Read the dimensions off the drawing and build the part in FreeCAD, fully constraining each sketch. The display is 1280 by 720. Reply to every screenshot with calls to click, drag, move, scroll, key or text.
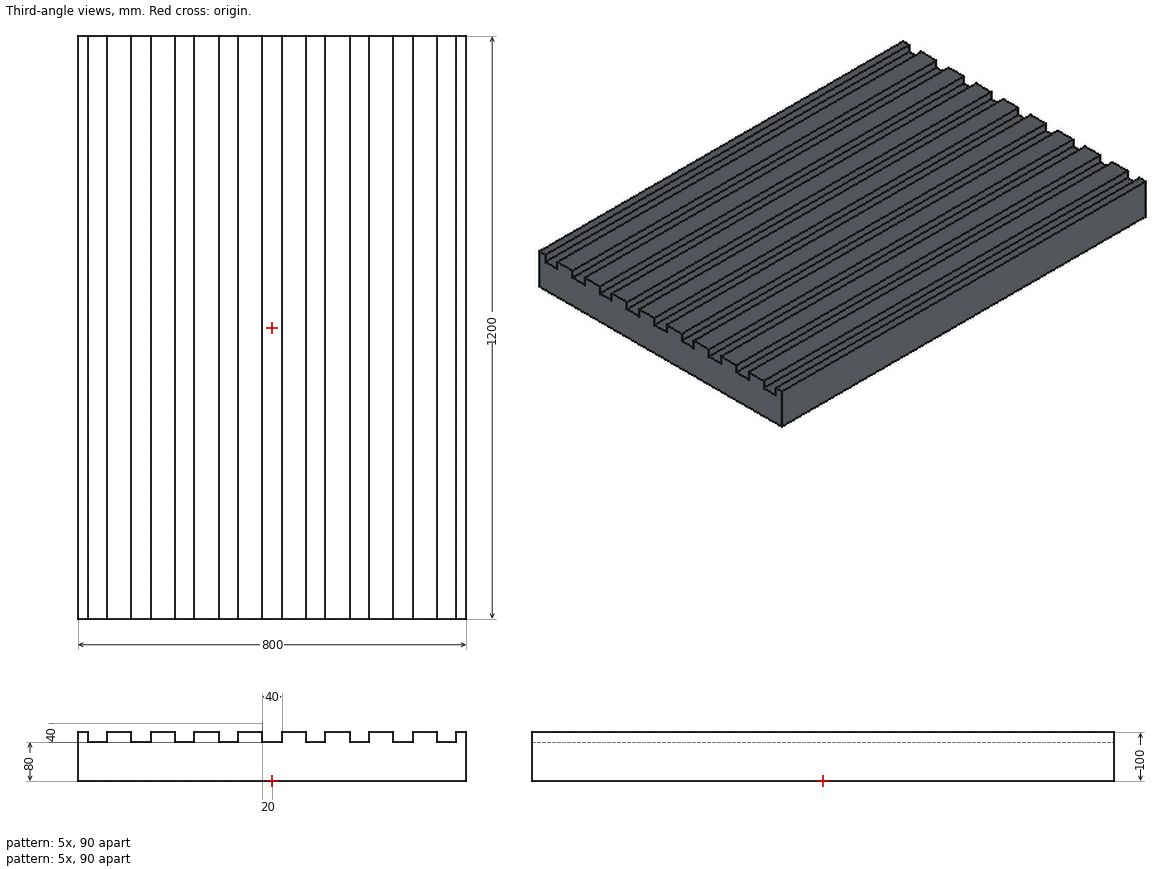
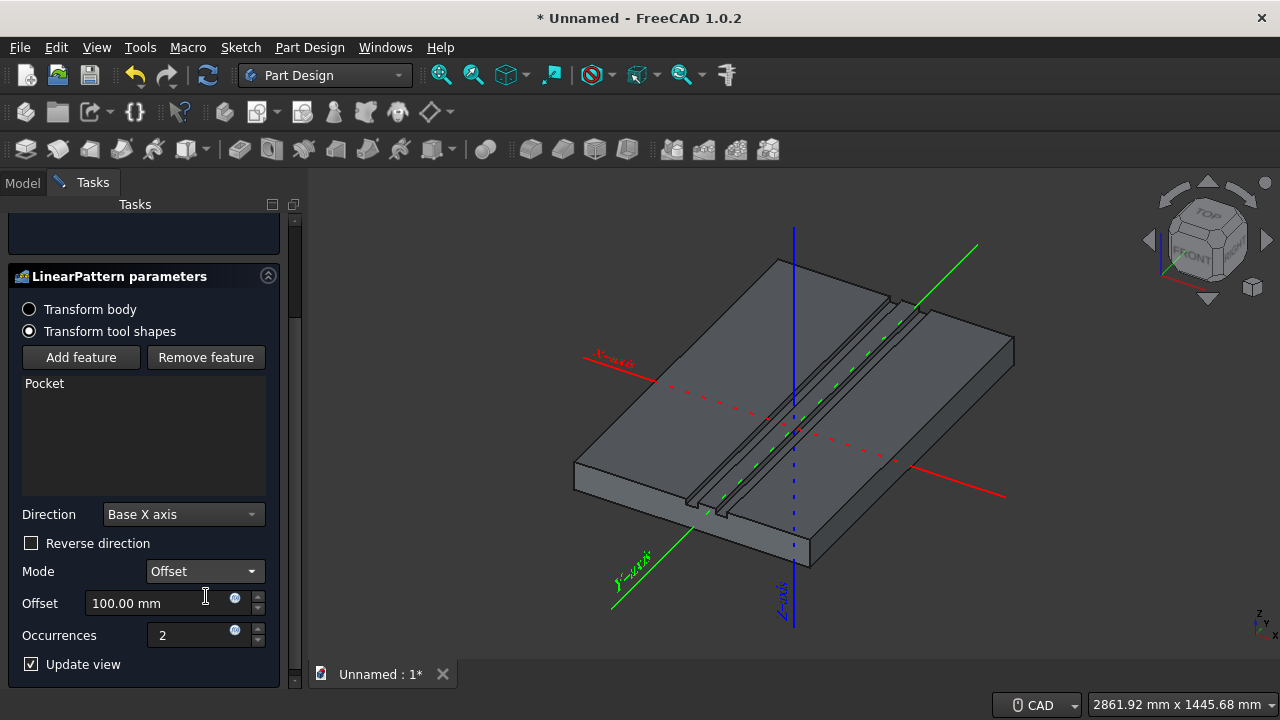
triple_click(168, 603)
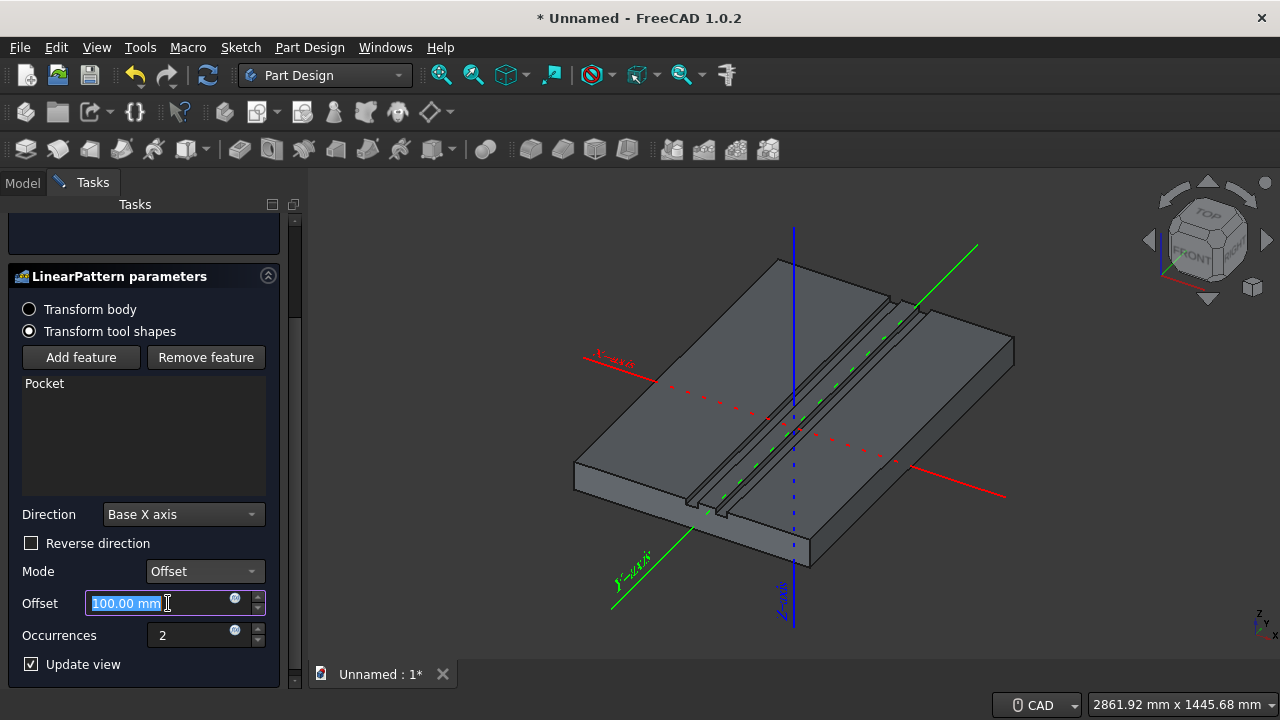
text(90)
key(Tab)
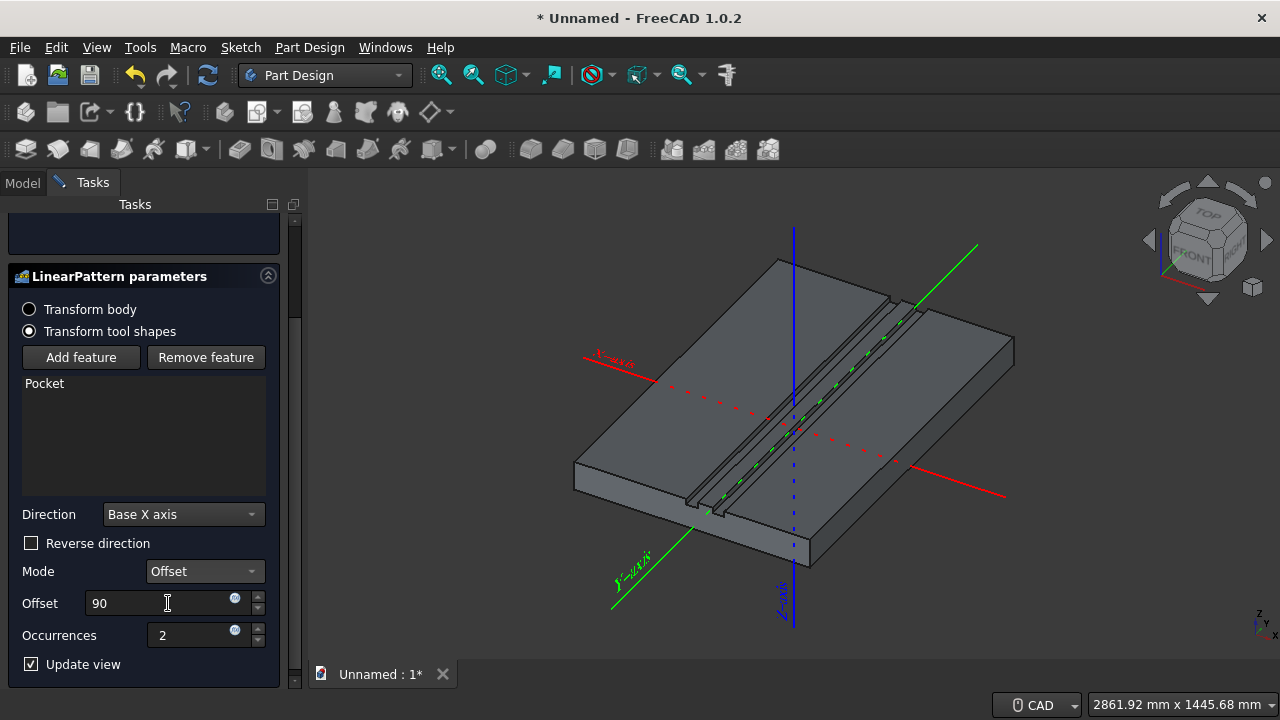
triple_click(198, 635)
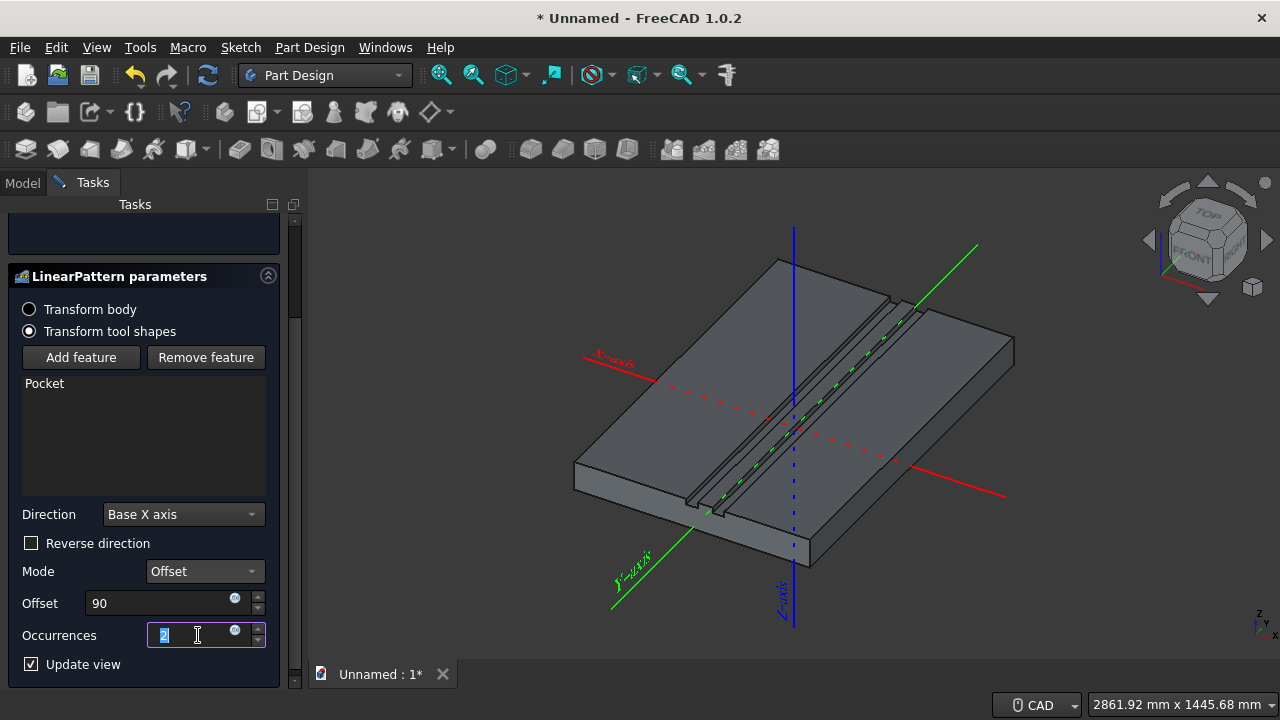
text(5)
key(Tab)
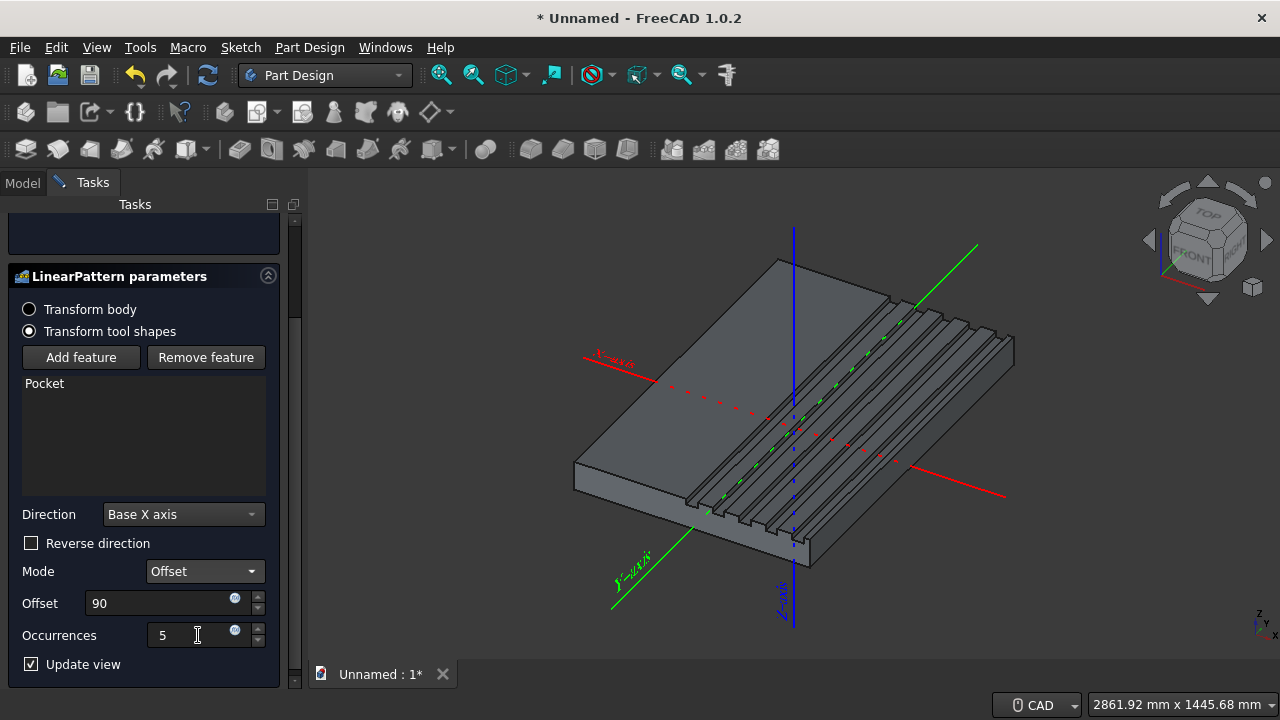
scroll(295, 451, up, 3)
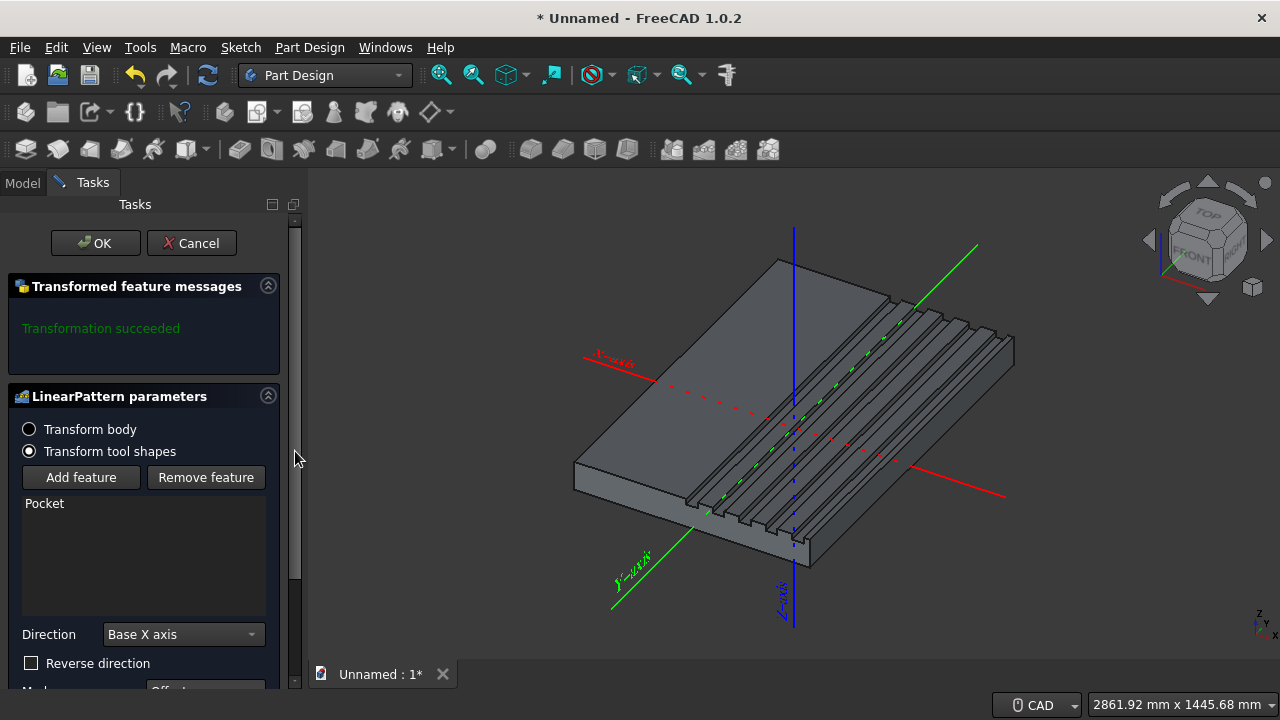
click(96, 243)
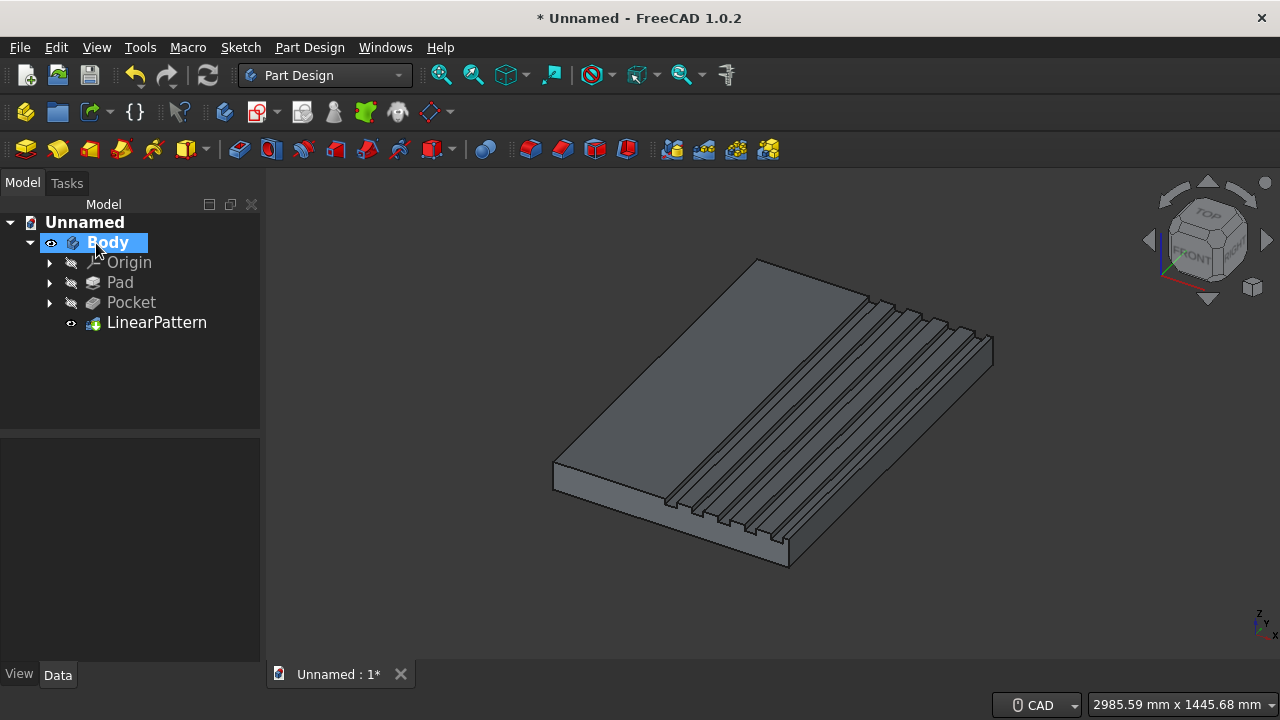
click(116, 303)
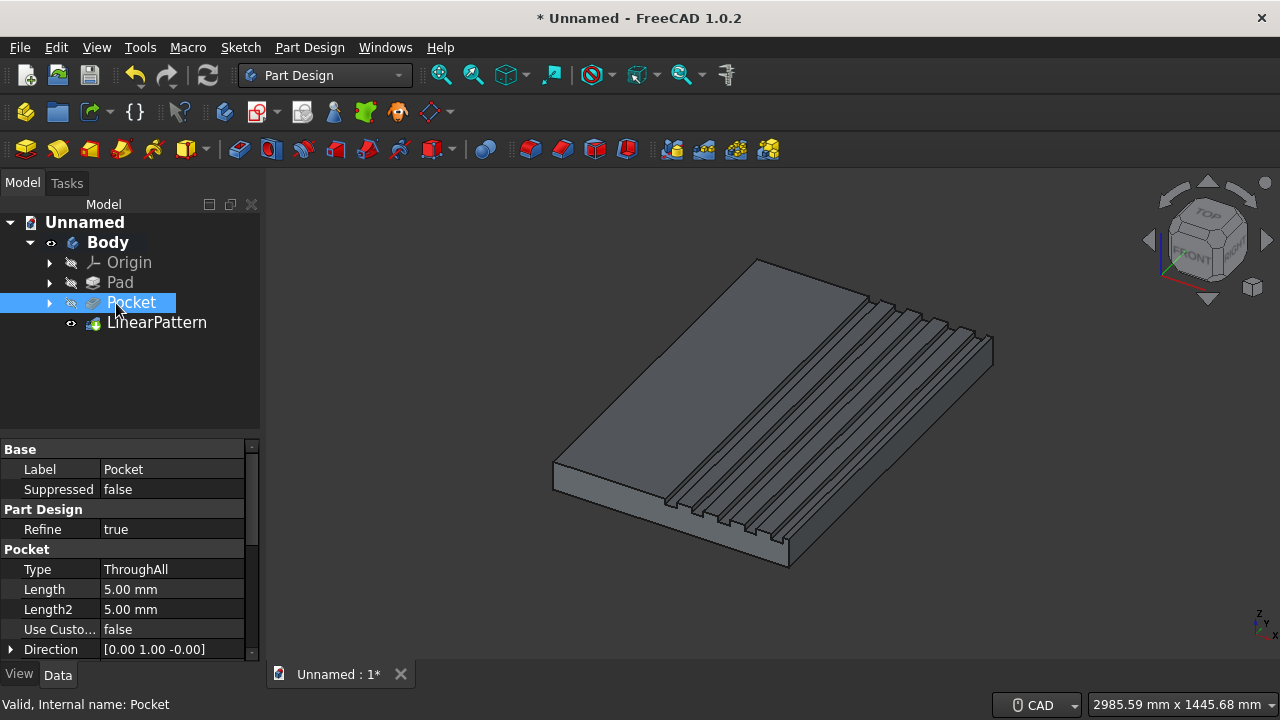
click(704, 150)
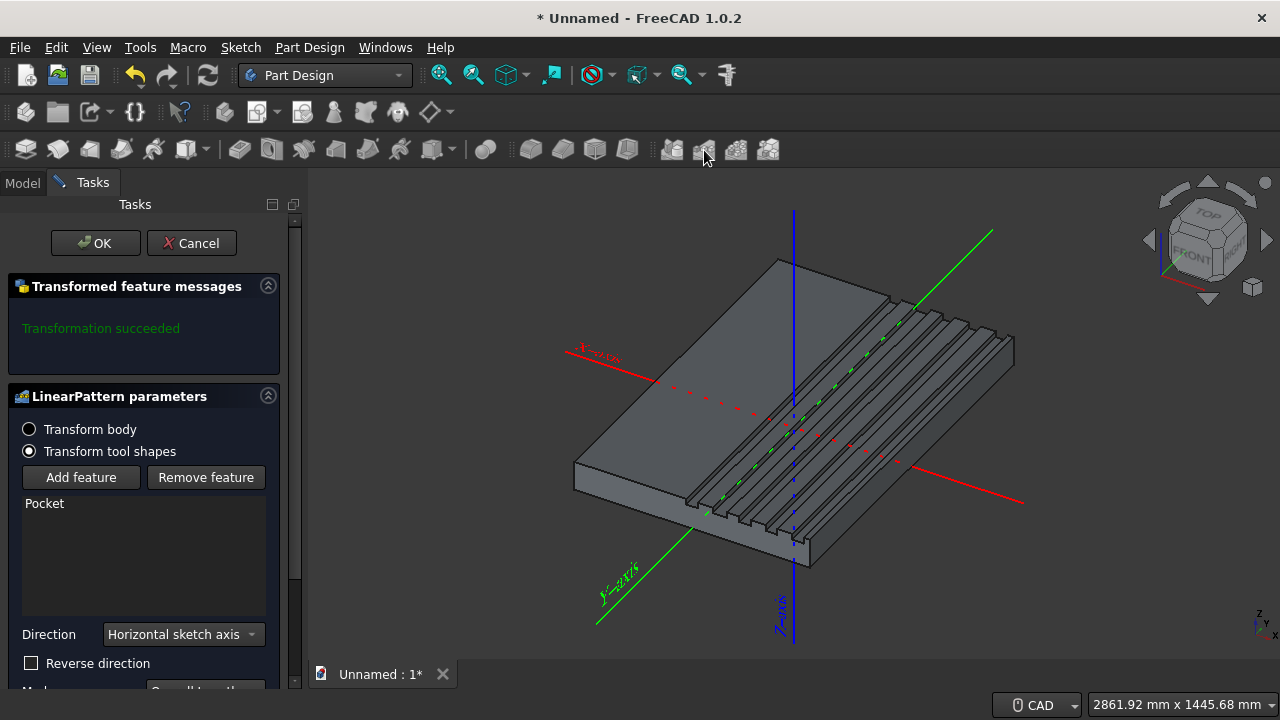
click(184, 634)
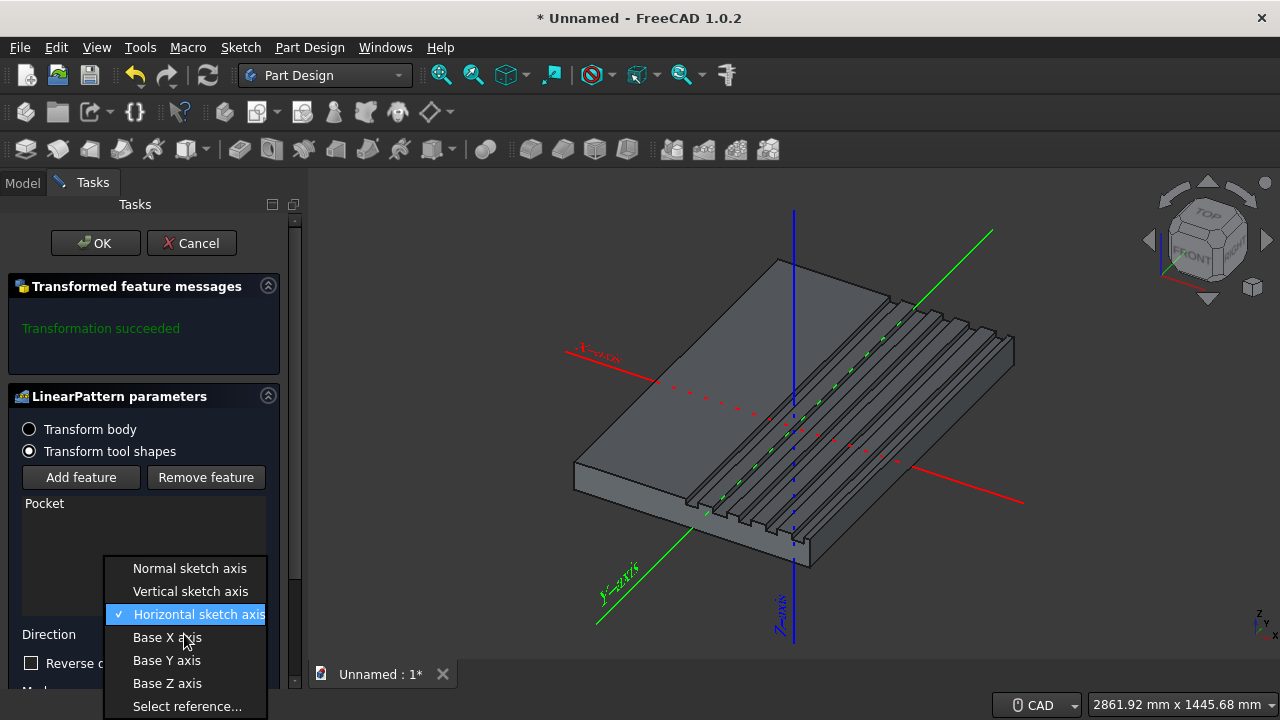
click(184, 638)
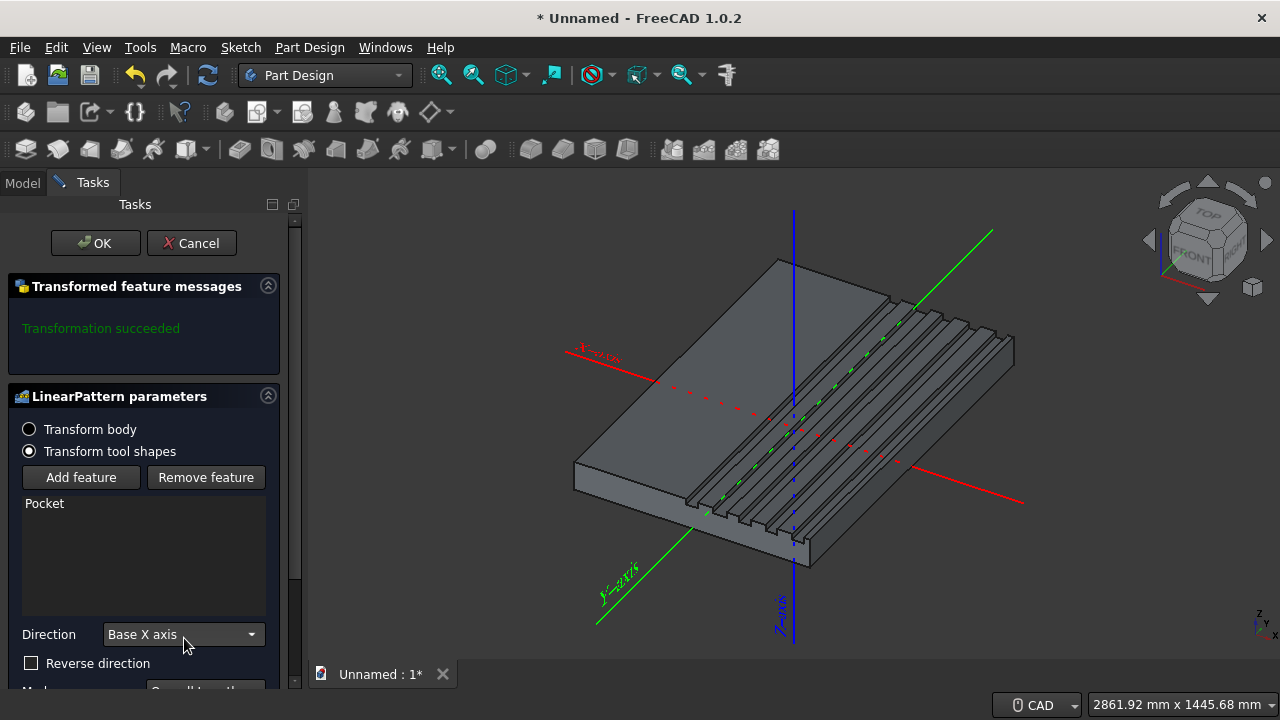
scroll(295, 451, down, 2)